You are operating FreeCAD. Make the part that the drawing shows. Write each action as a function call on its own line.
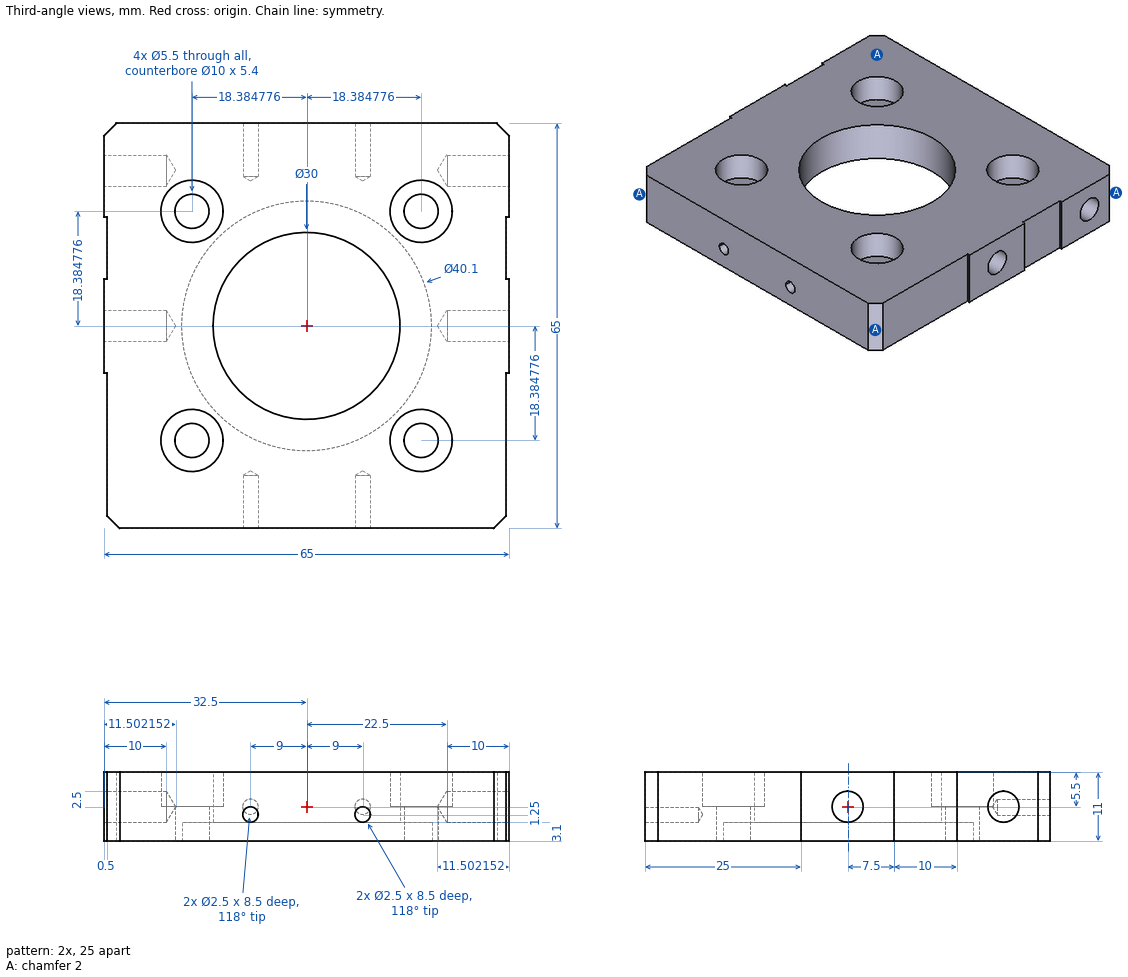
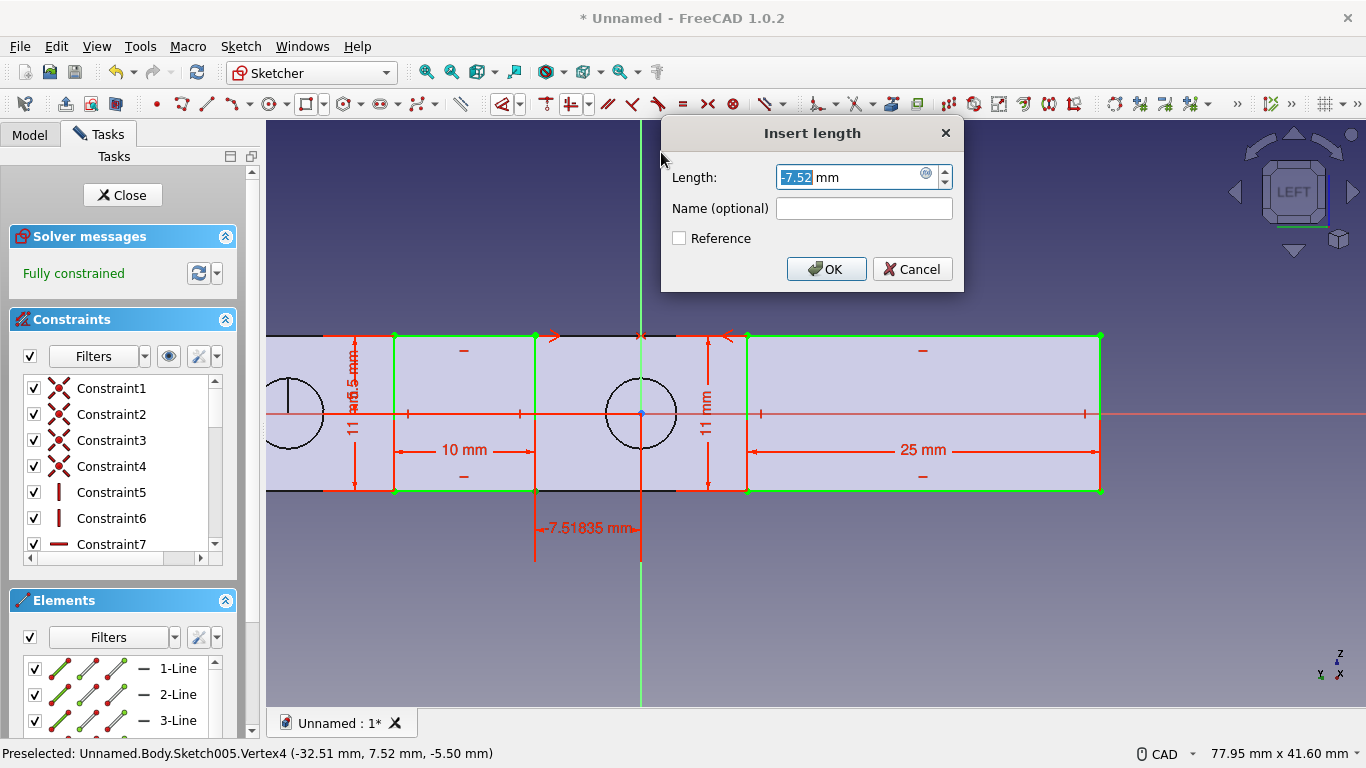
text(-7.5)
key(Return)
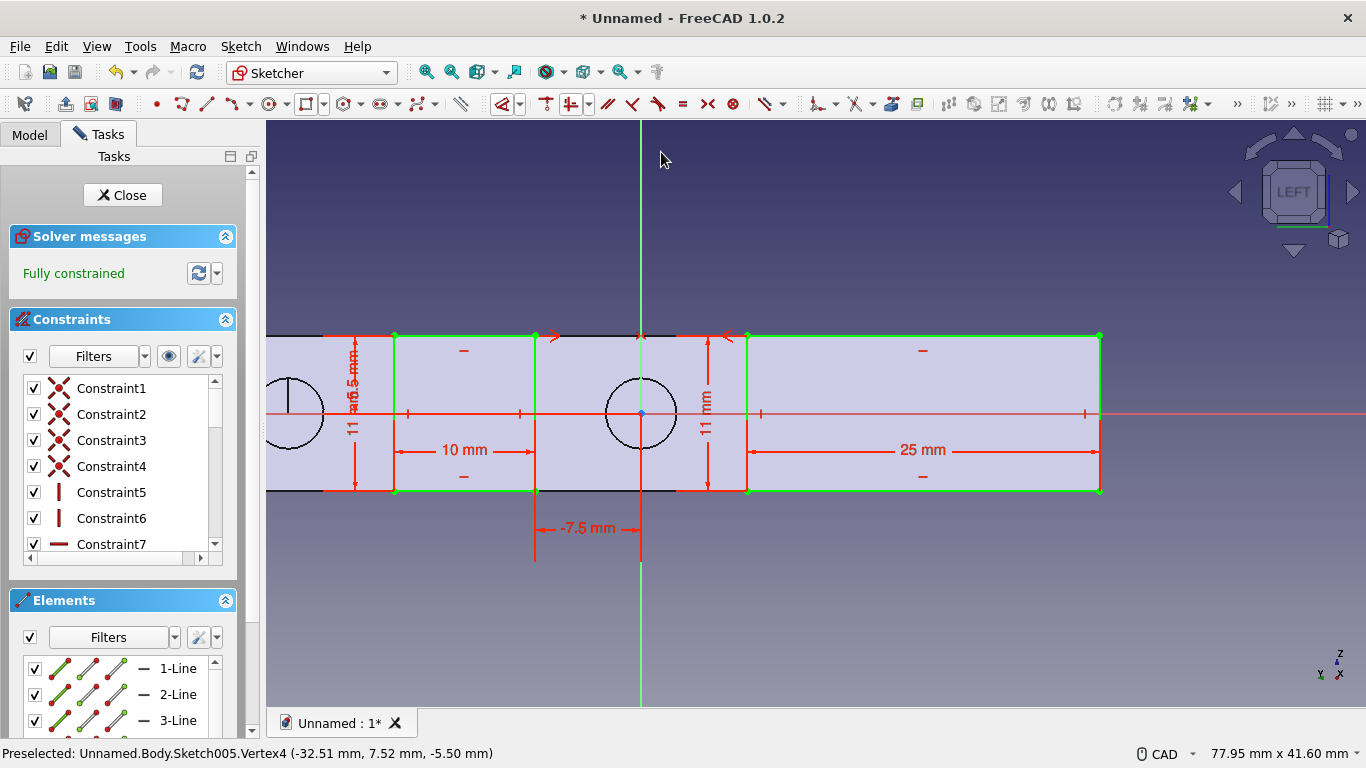
click(123, 195)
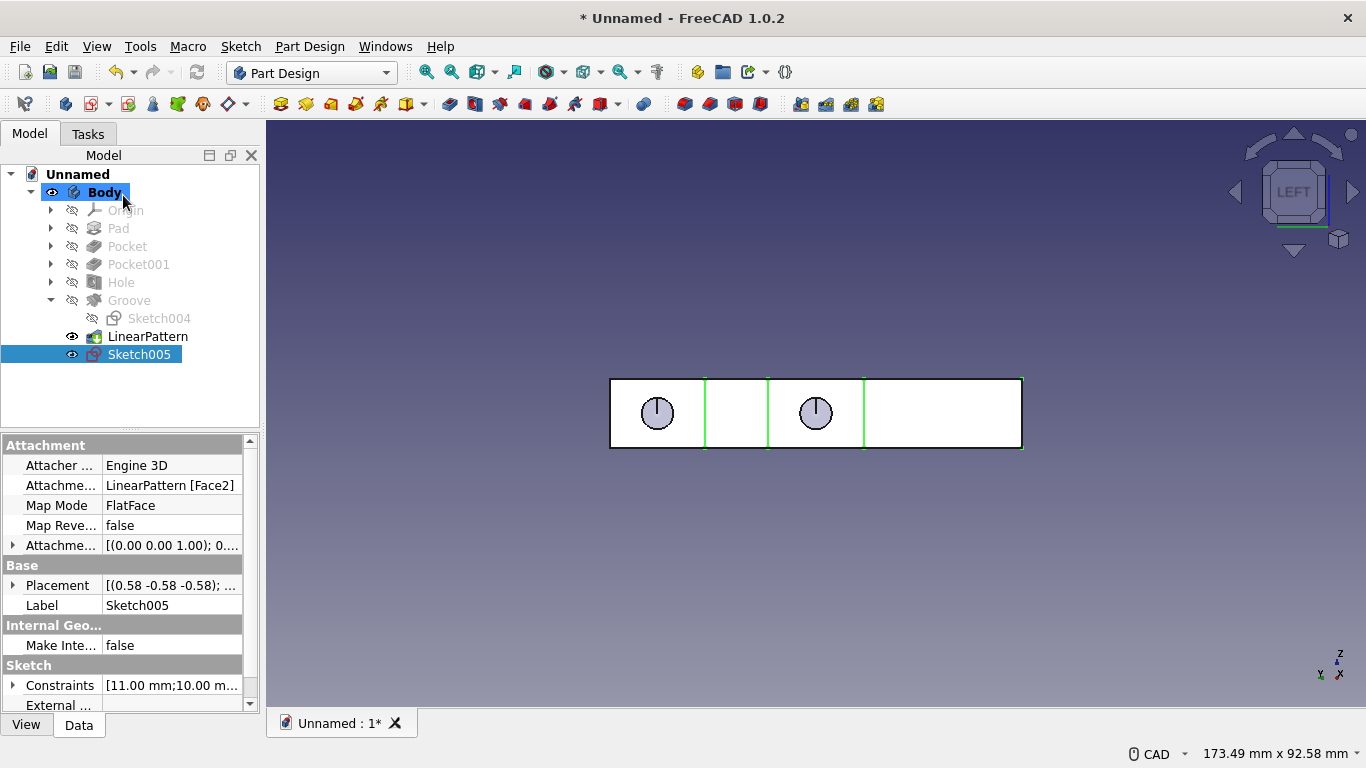
click(450, 104)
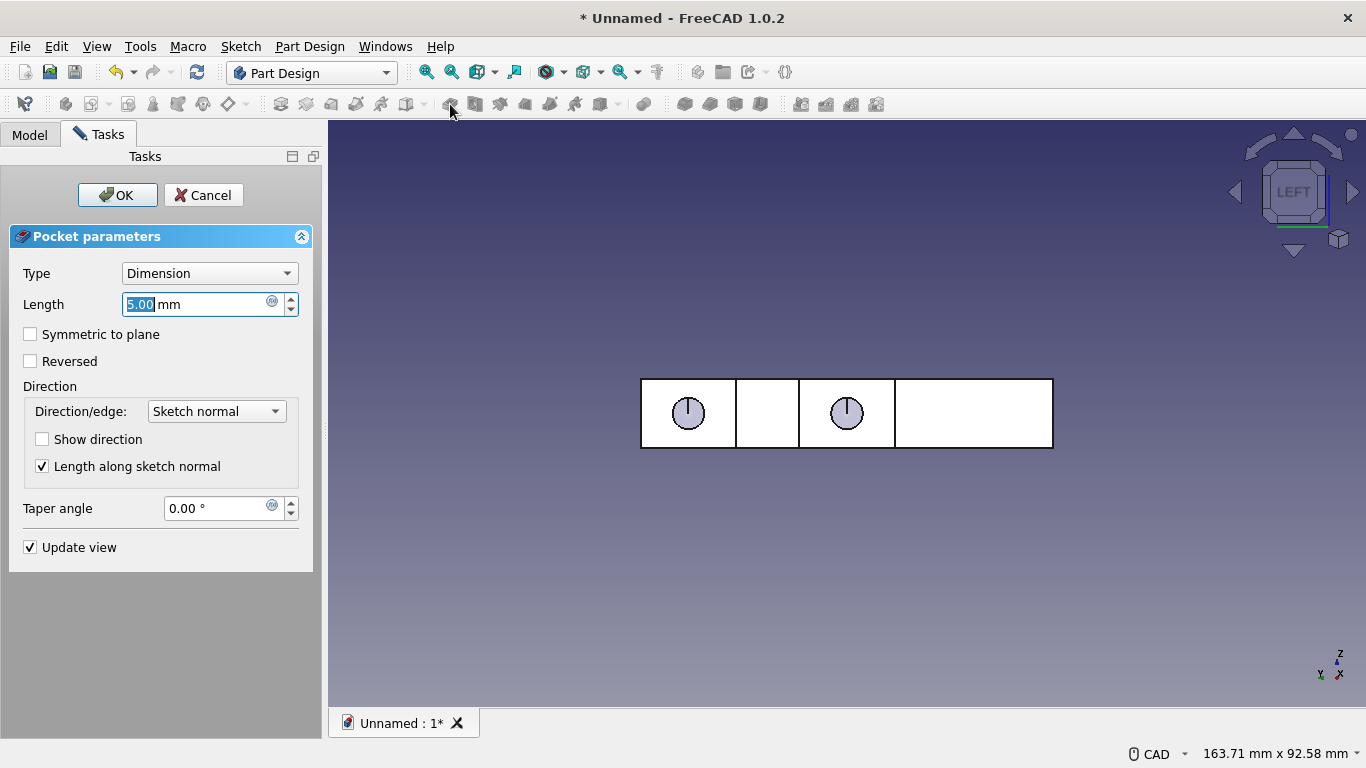
text(0.5)
key(Tab)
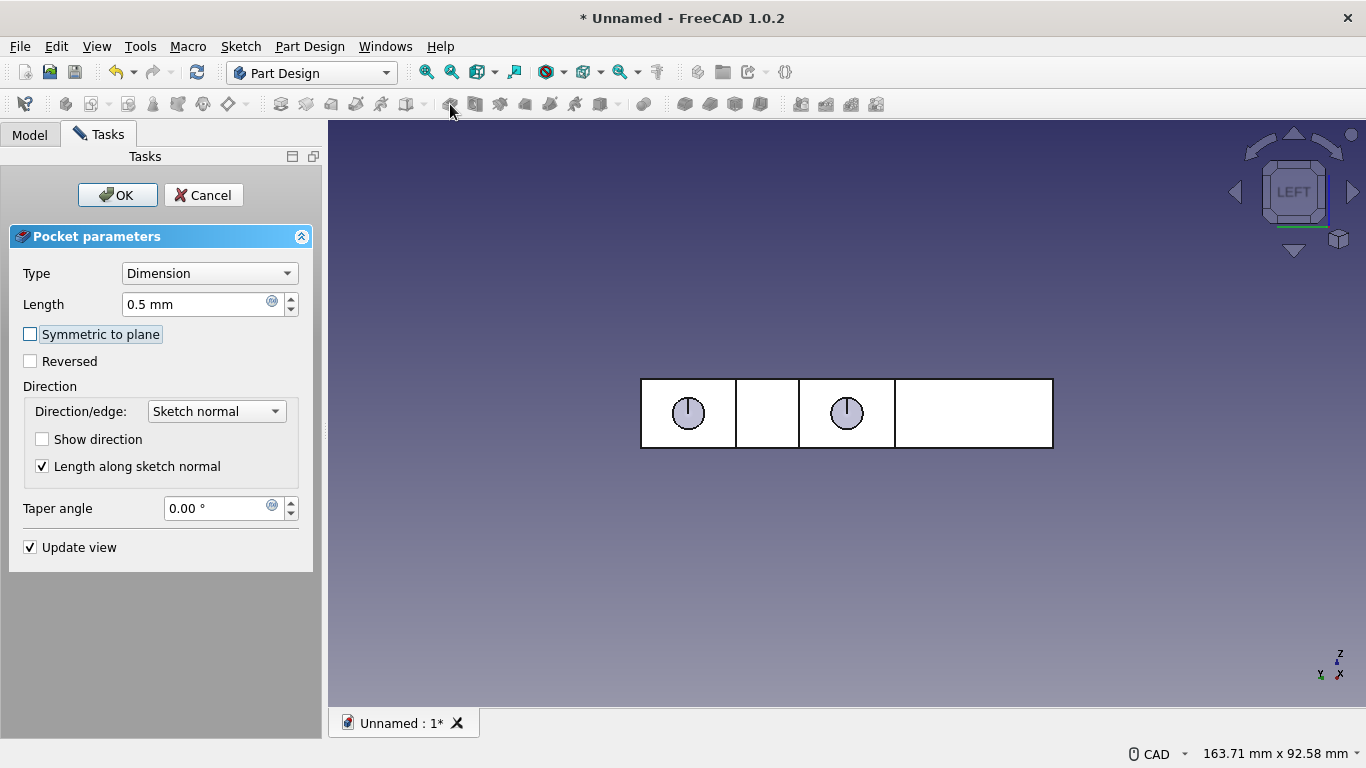
click(118, 195)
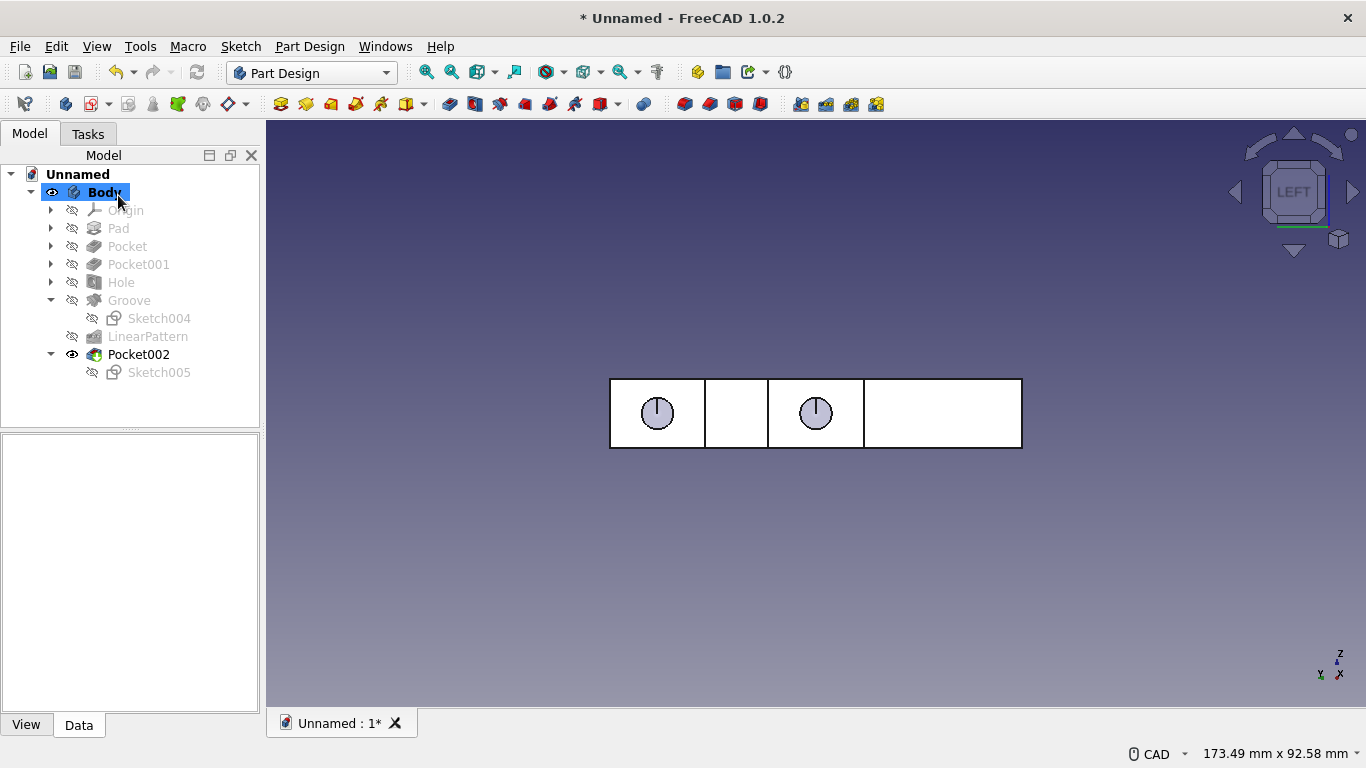
click(427, 72)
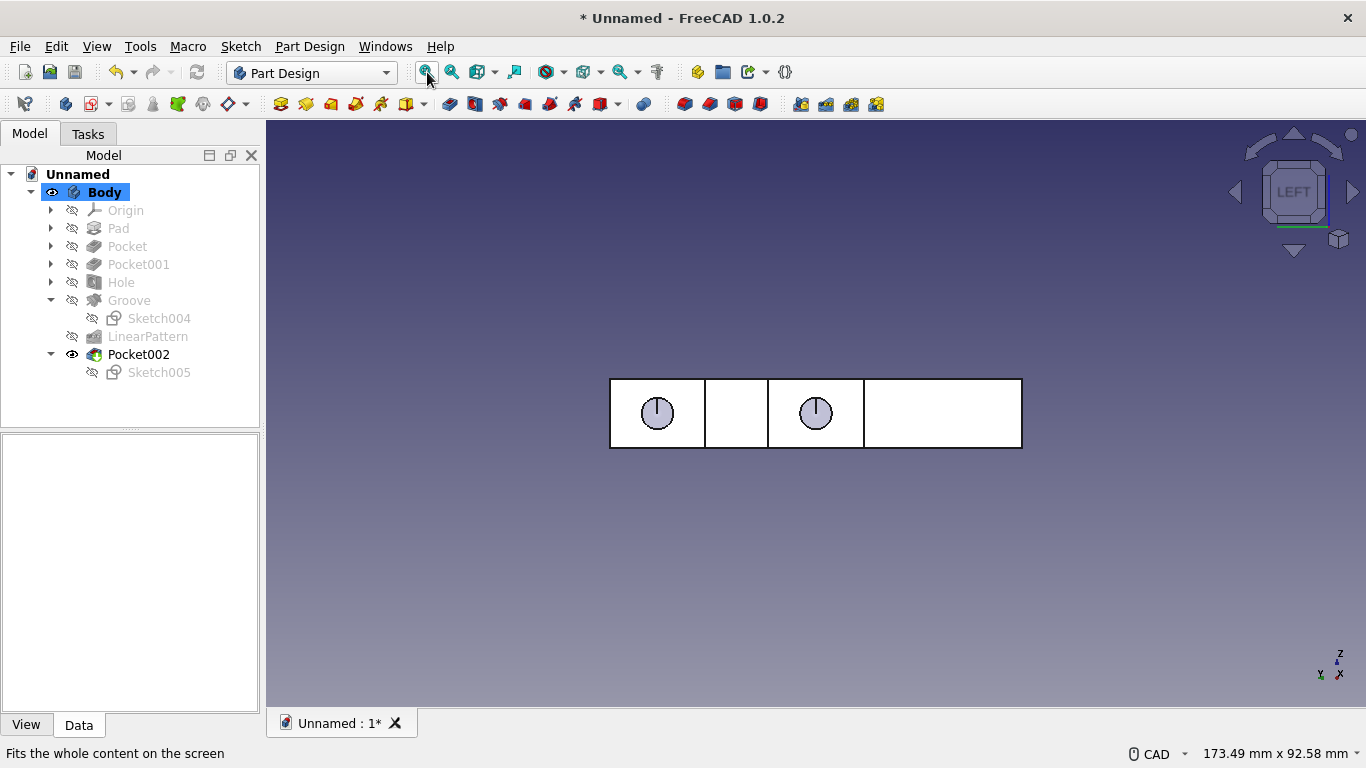
click(117, 300)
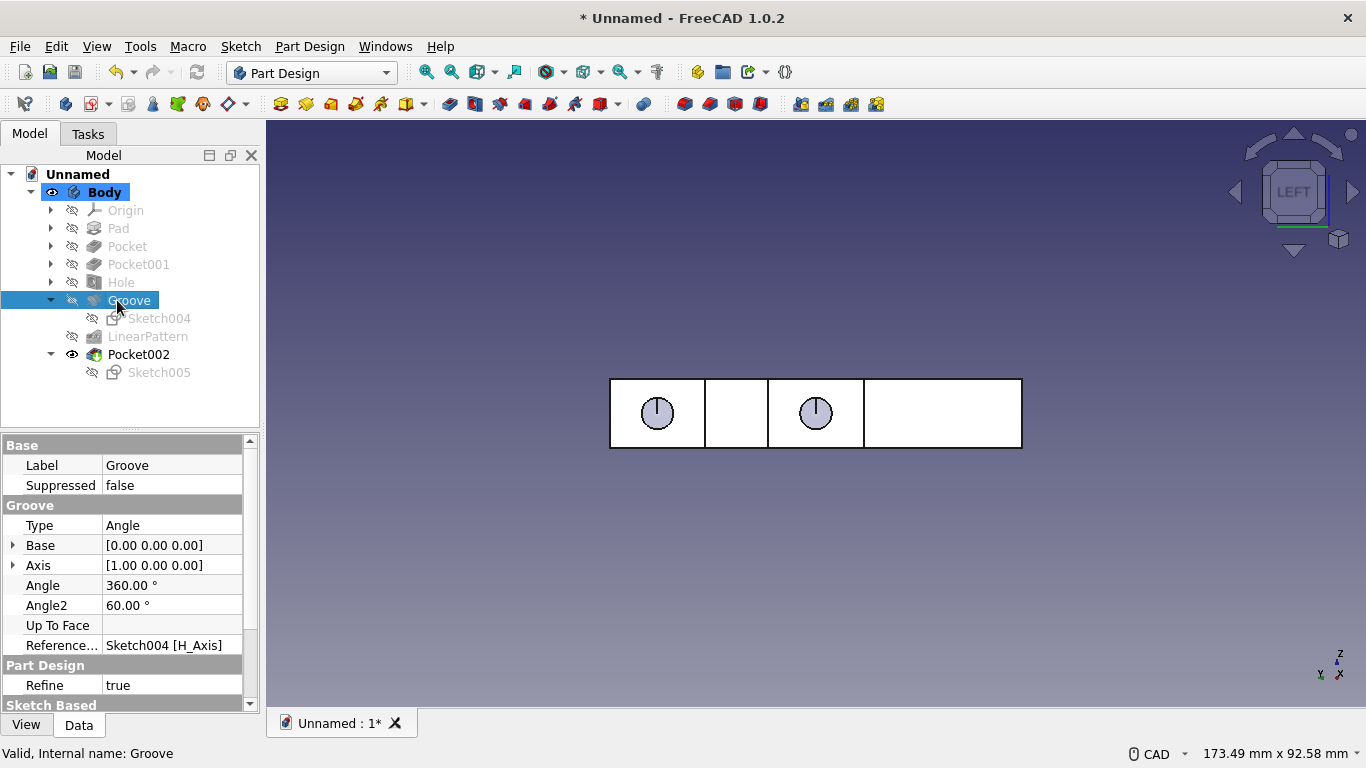
click(117, 354, ctrl)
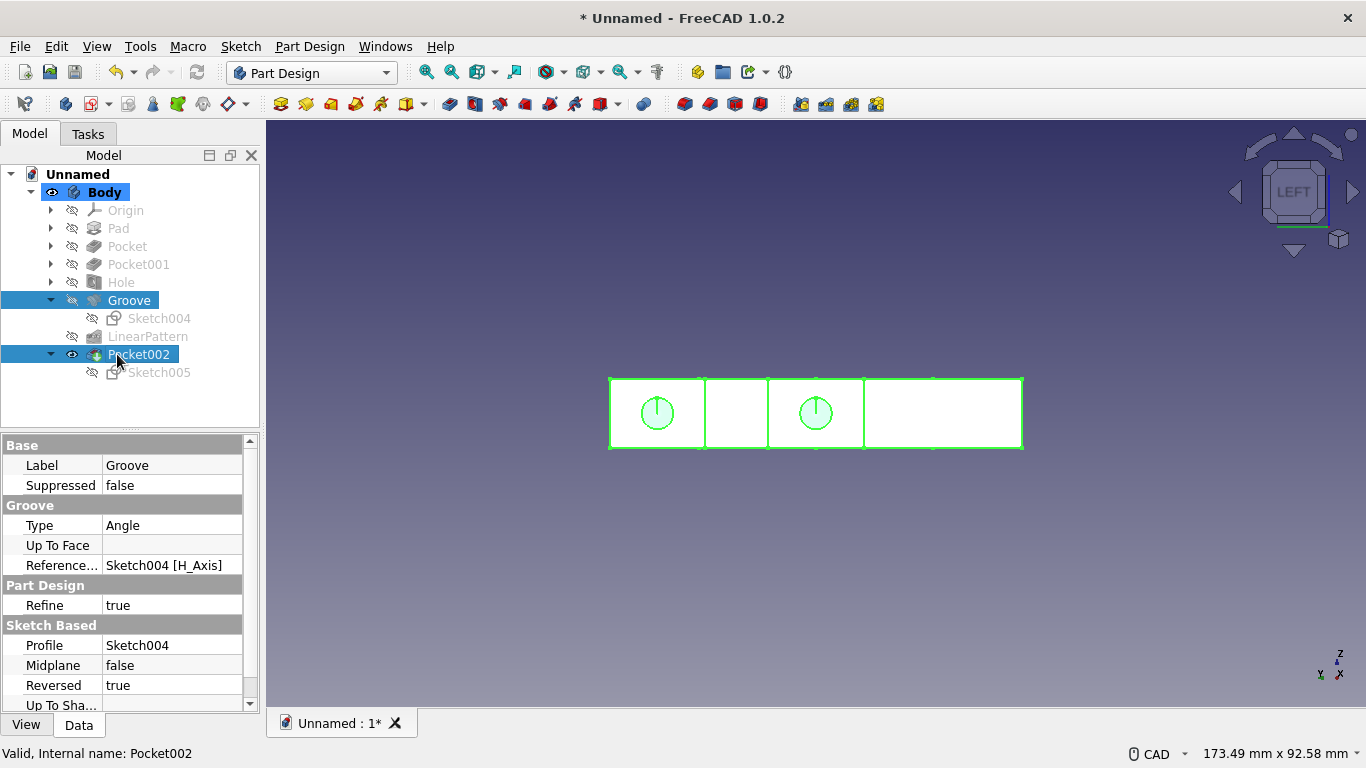
click(801, 104)